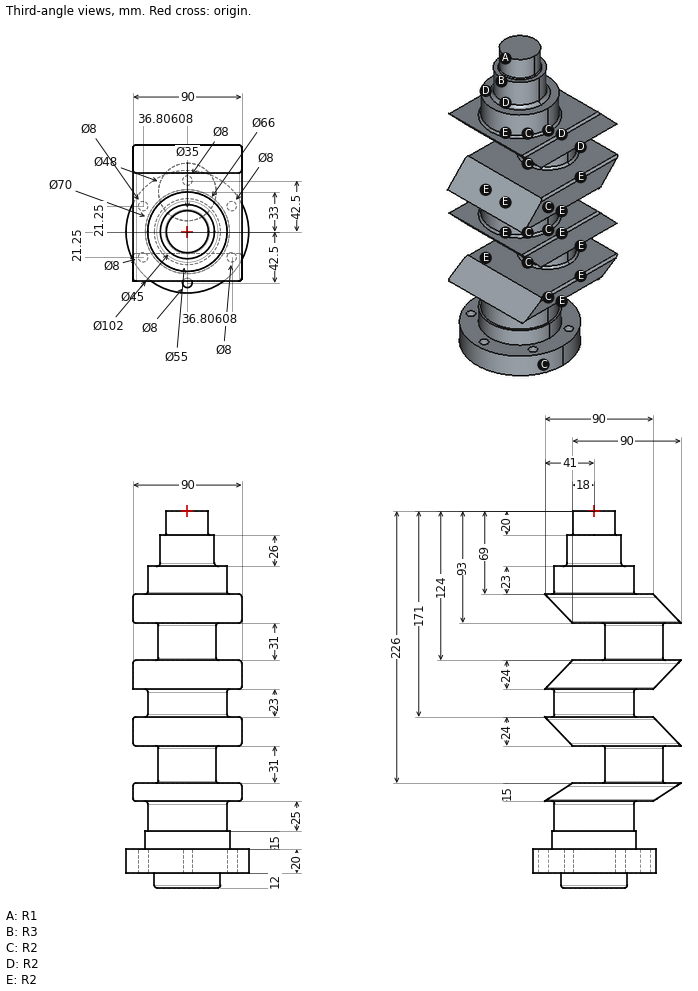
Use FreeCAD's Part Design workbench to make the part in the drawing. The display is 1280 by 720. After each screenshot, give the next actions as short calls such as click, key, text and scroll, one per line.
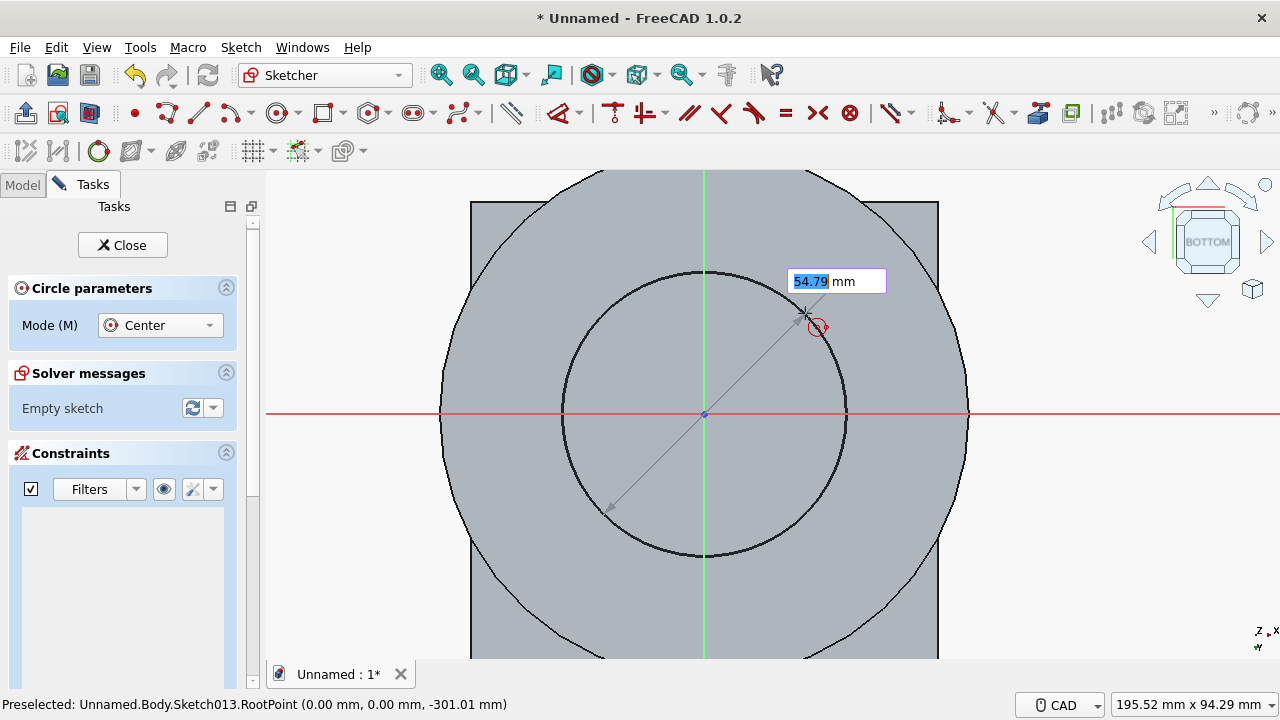
text(55)
key(Return)
key(Escape)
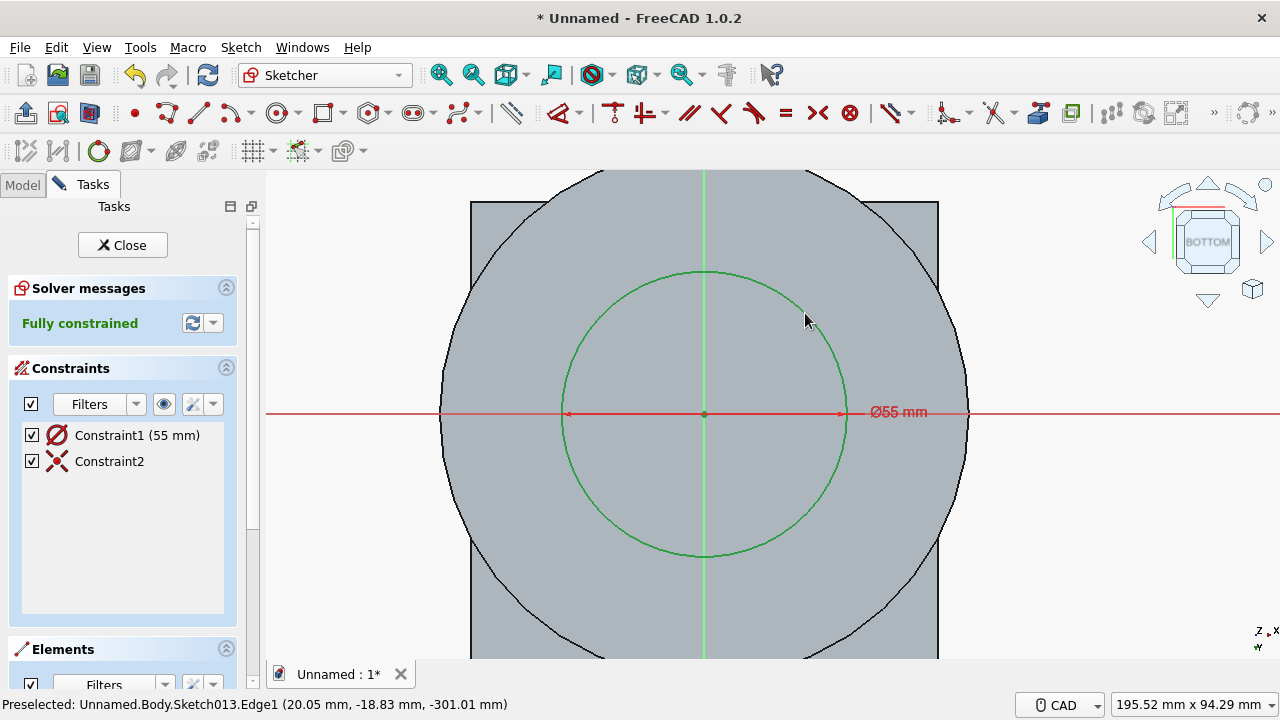
click(123, 245)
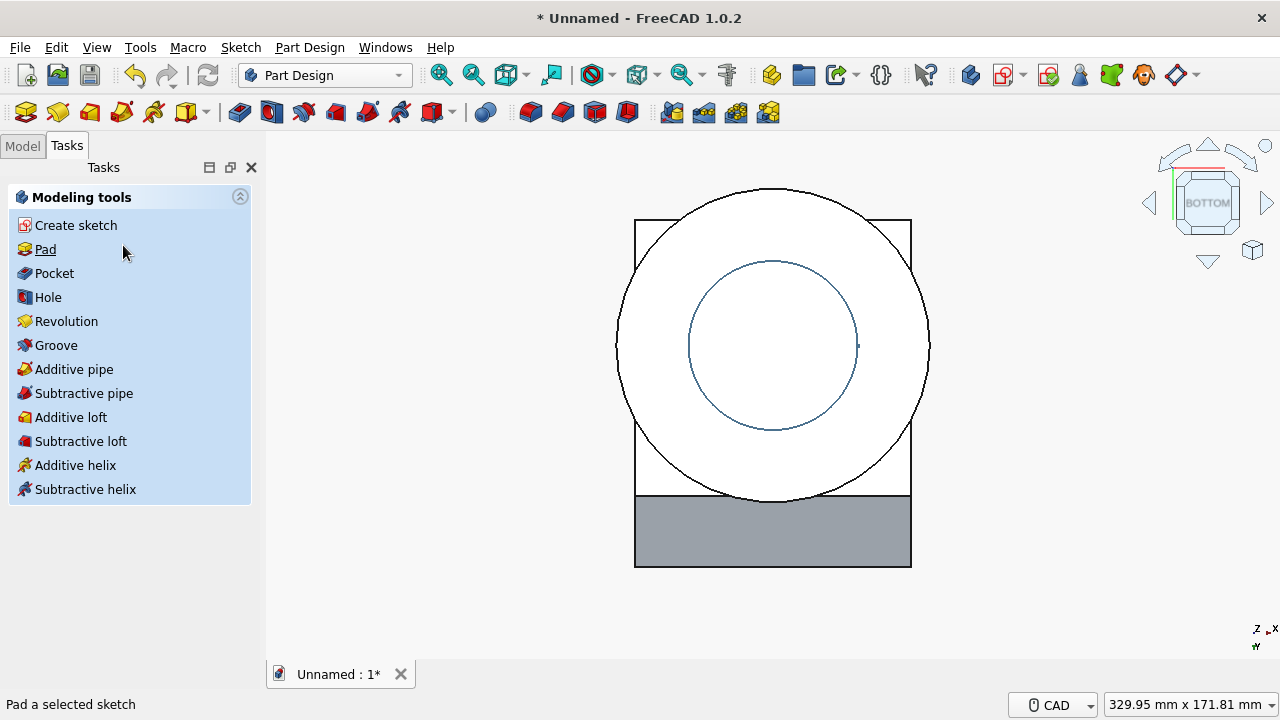
click(26, 112)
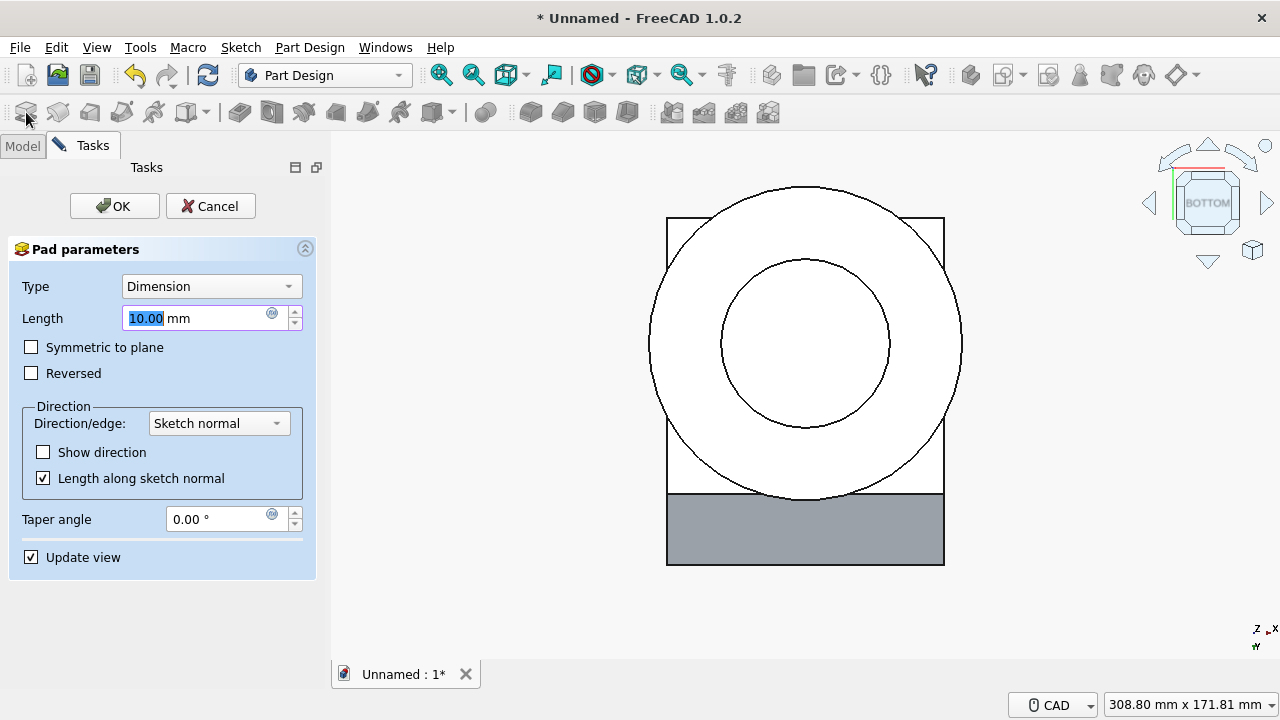
text(12)
key(Tab)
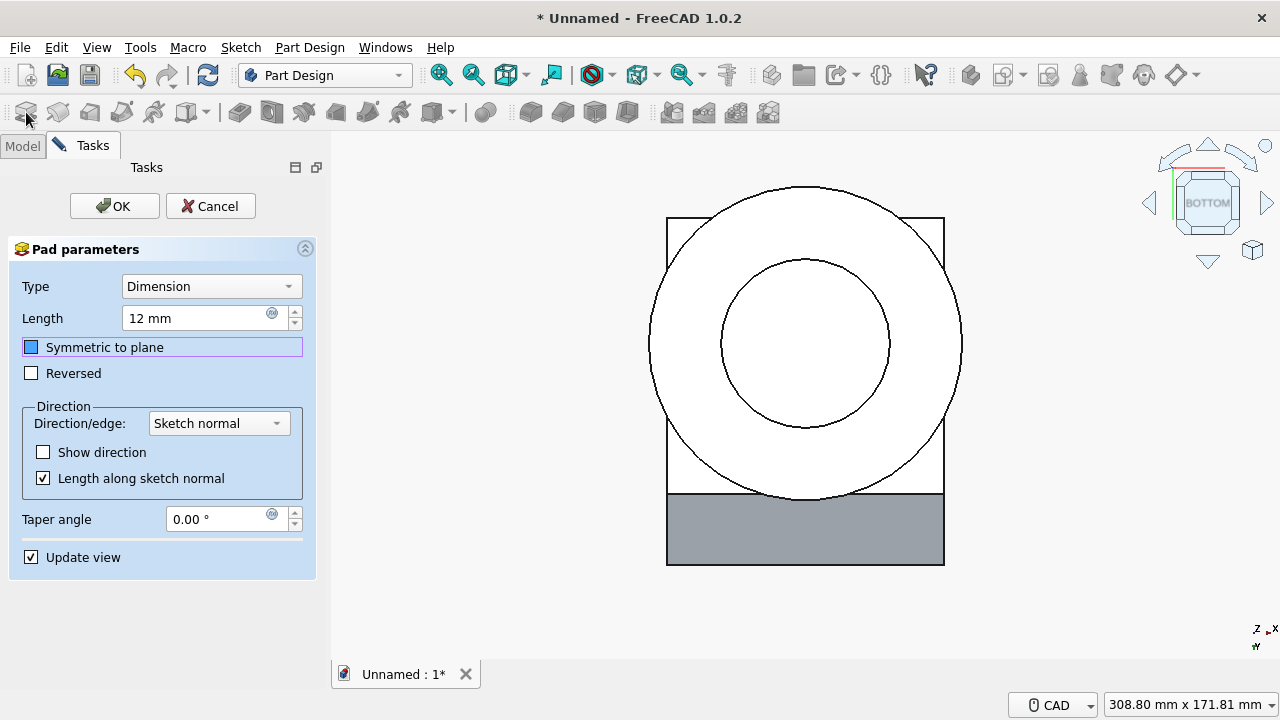
click(115, 206)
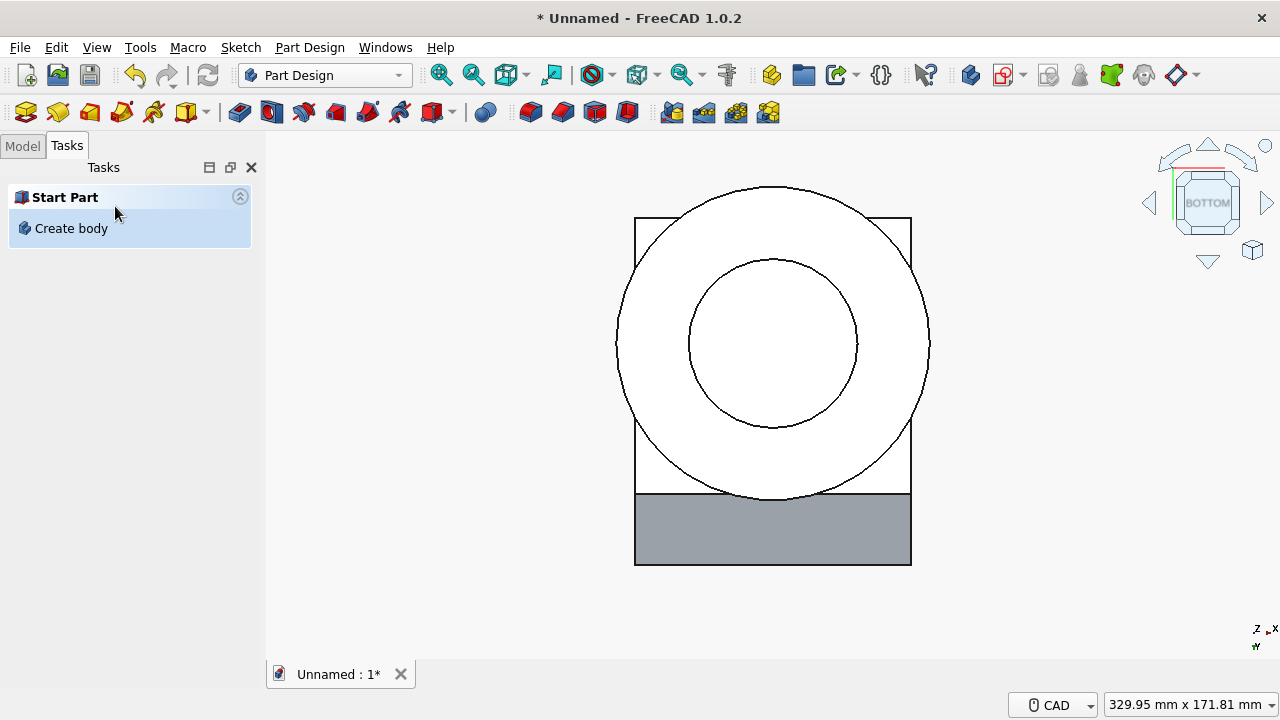
click(863, 432)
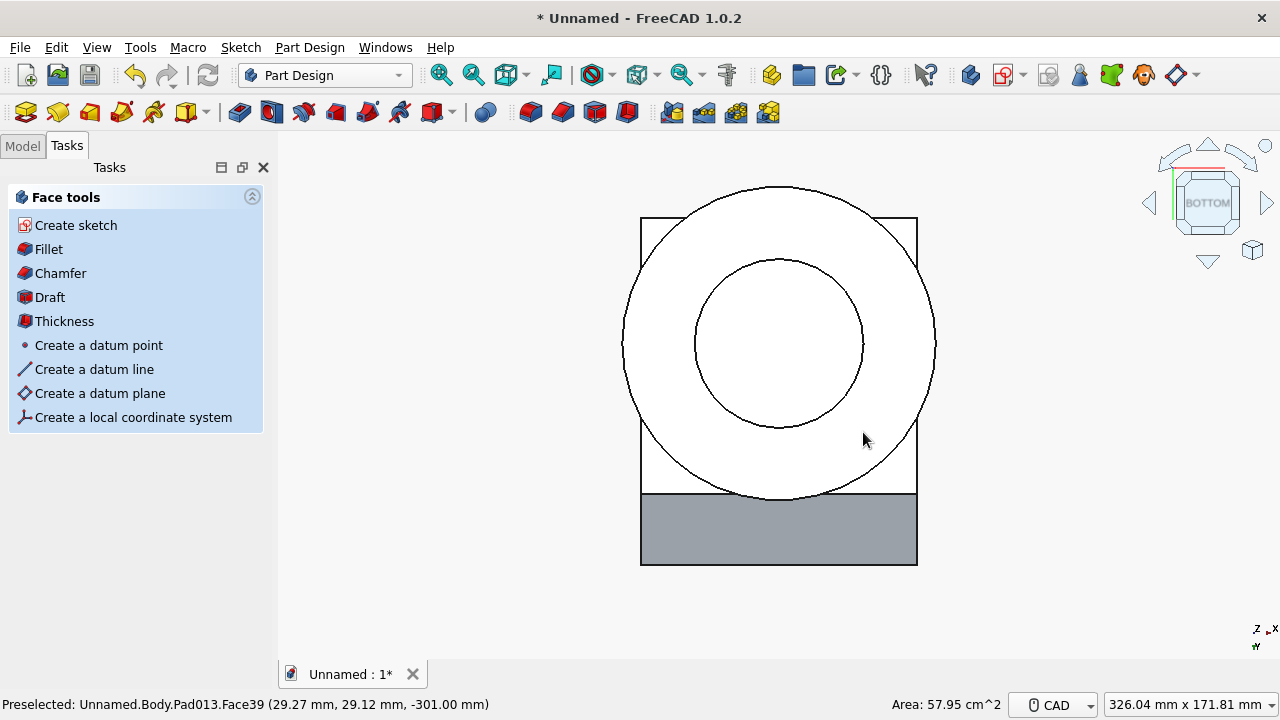
click(1004, 76)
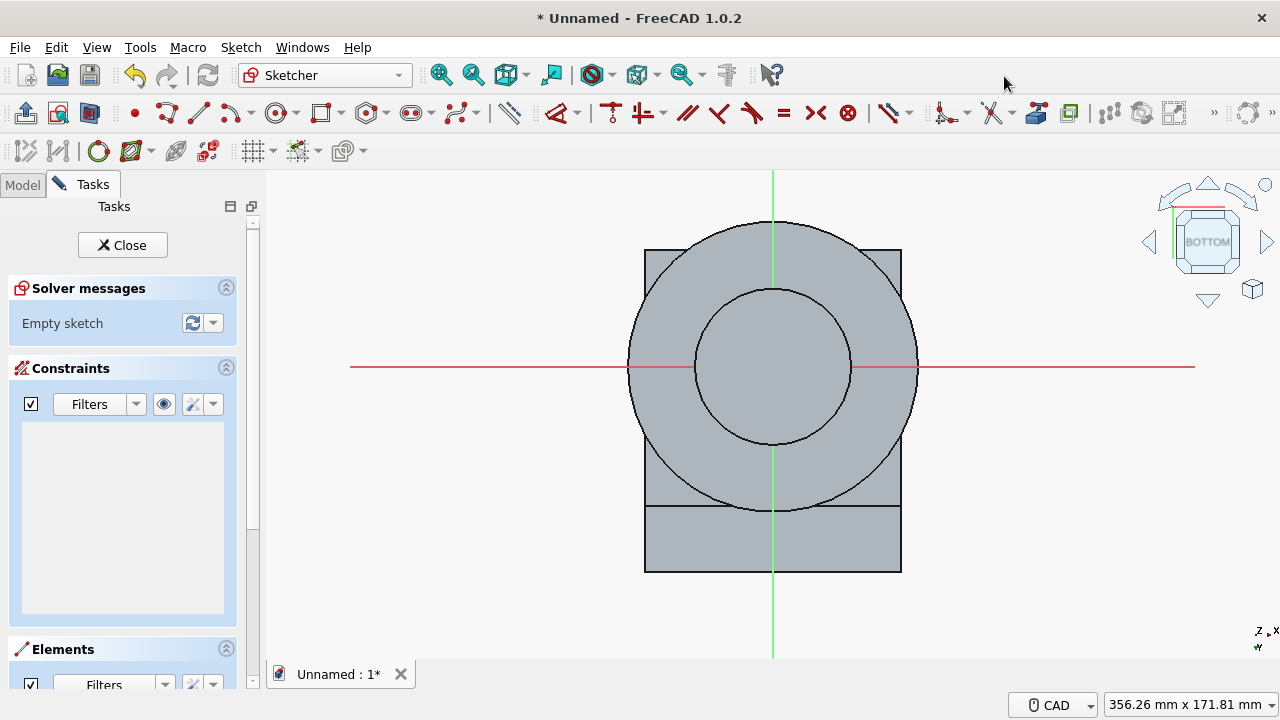
click(90, 114)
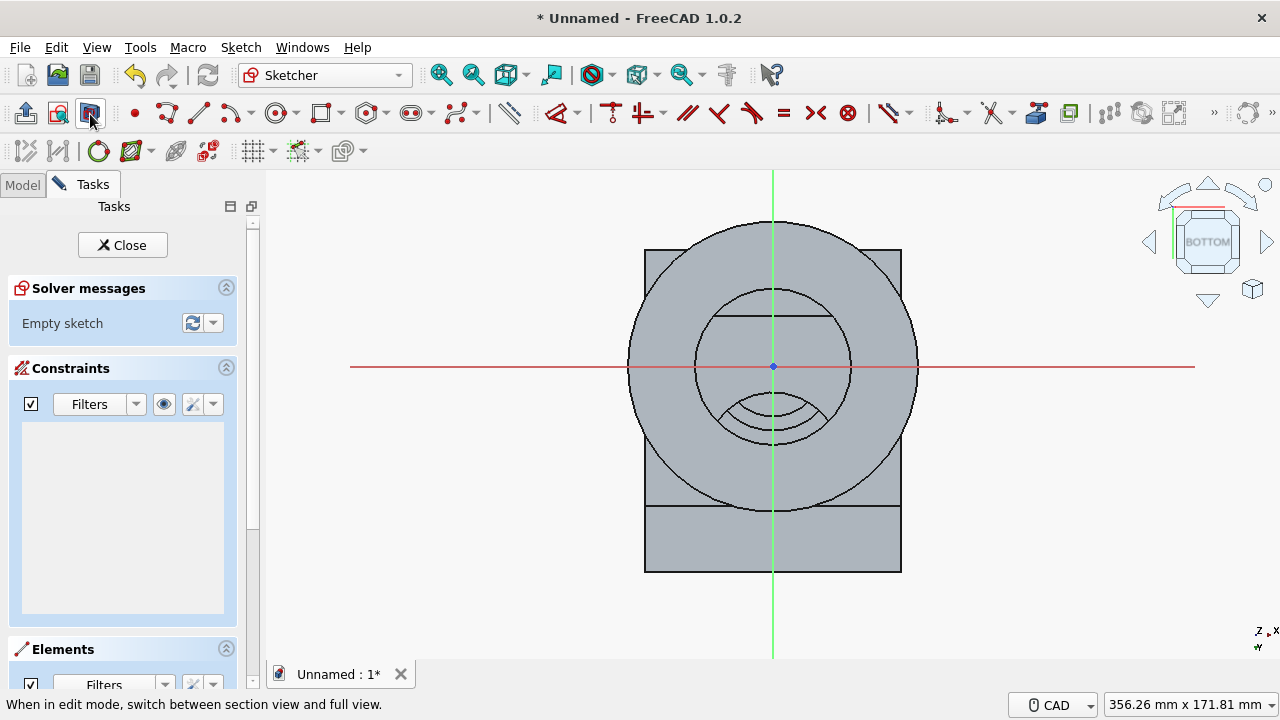
scroll(779, 494, up, 13)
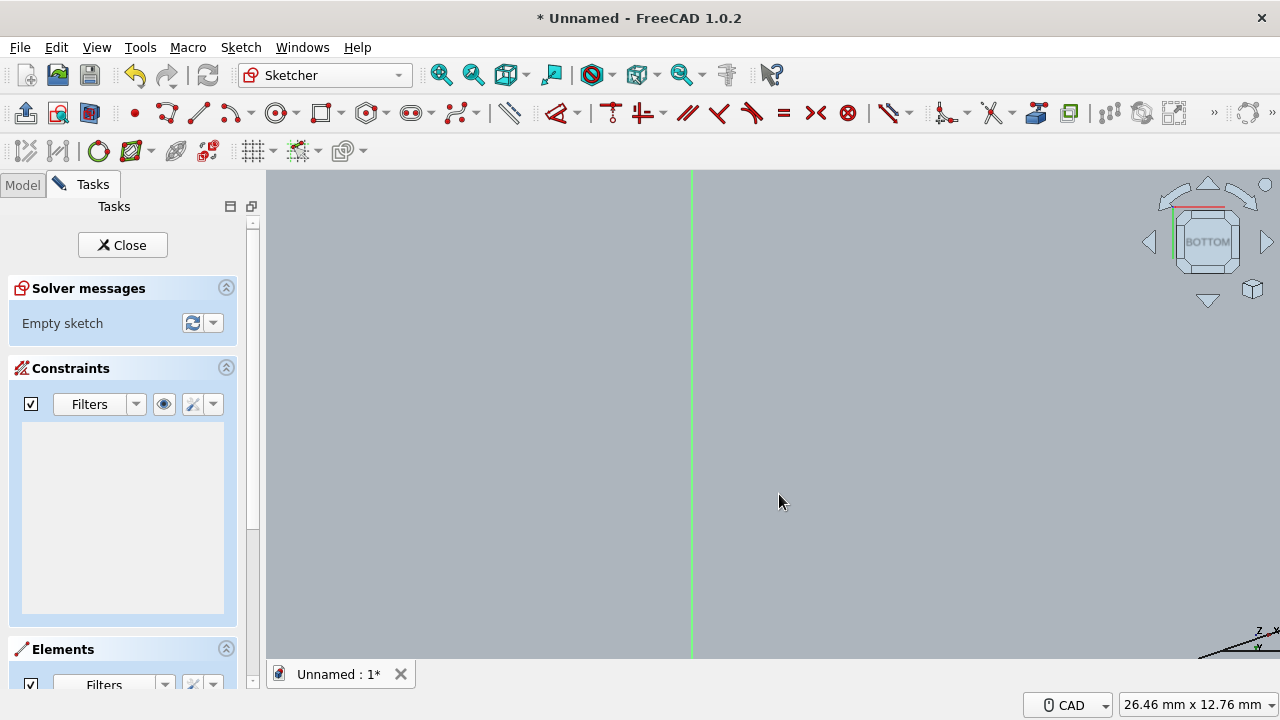
click(276, 114)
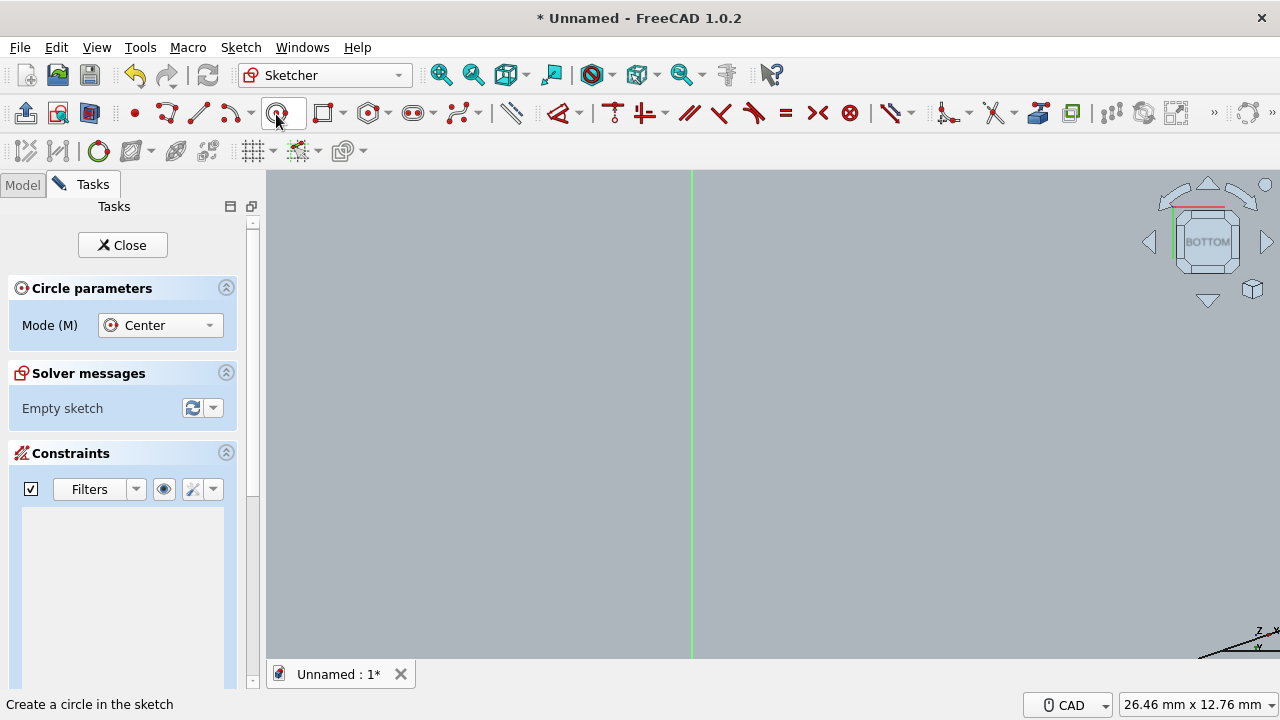
click(692, 402)
move(801, 293)